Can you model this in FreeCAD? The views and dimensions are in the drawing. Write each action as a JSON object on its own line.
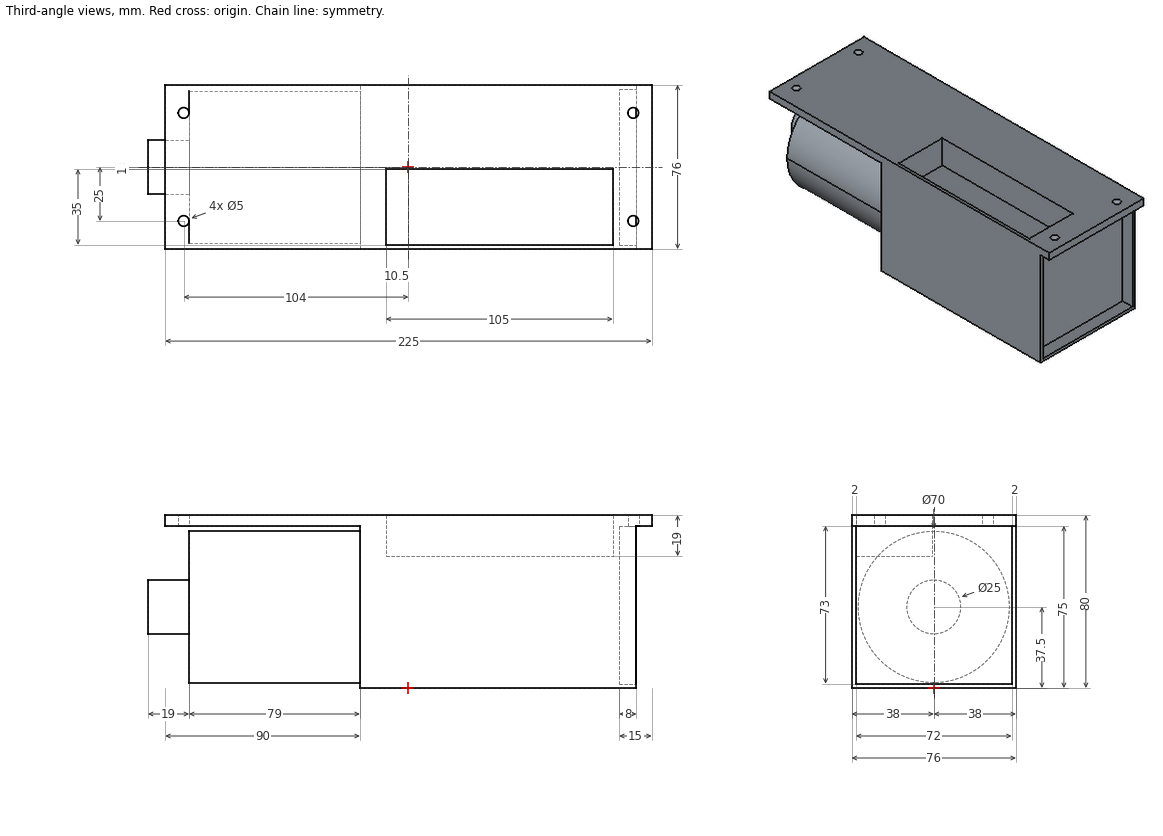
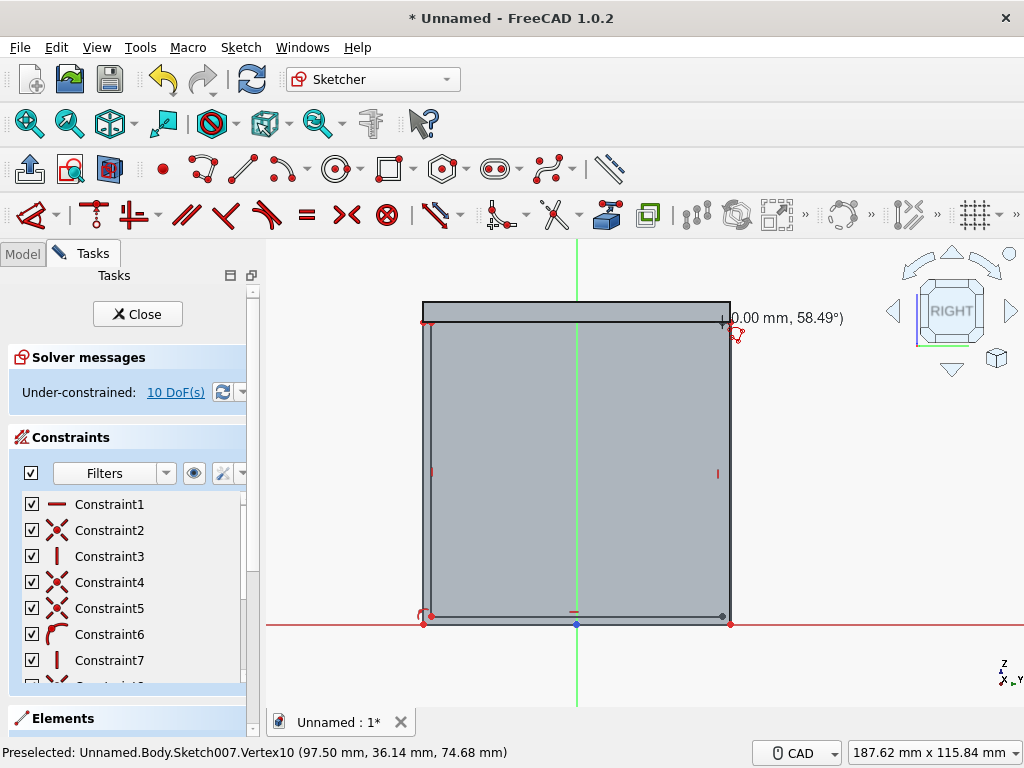
{"action": "scroll", "coordinate": [722, 617], "scroll_direction": "up", "scroll_amount": 4}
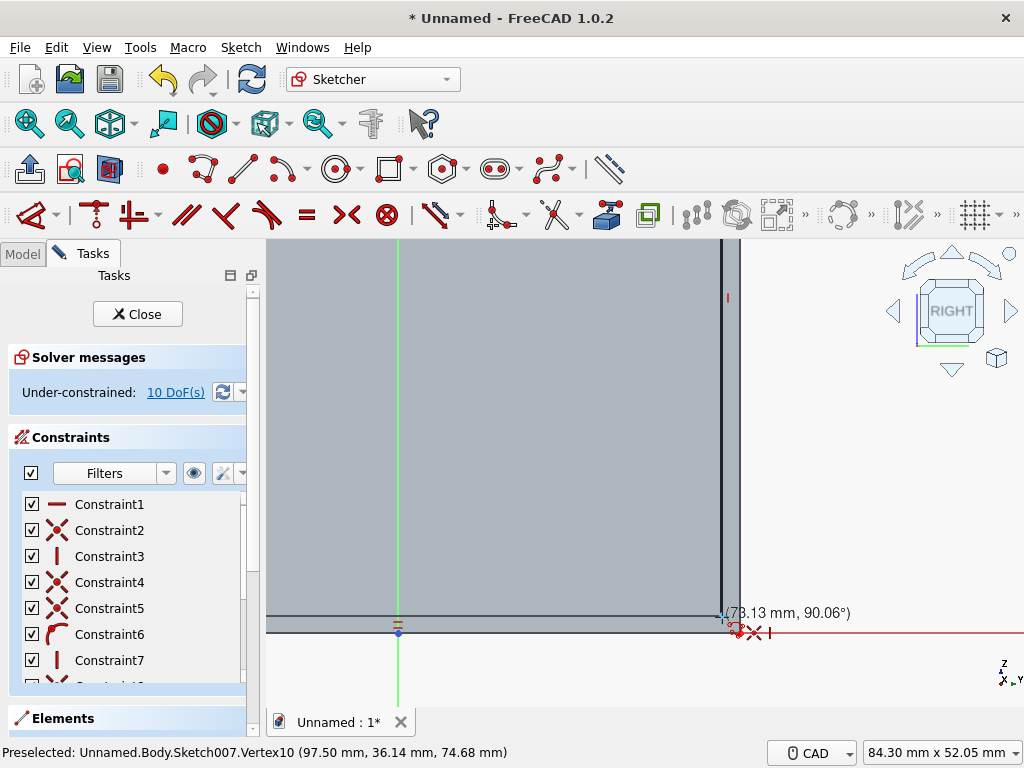
{"action": "left_click", "coordinate": [722, 616]}
{"action": "key", "text": "Escape"}
{"action": "key", "text": "Escape"}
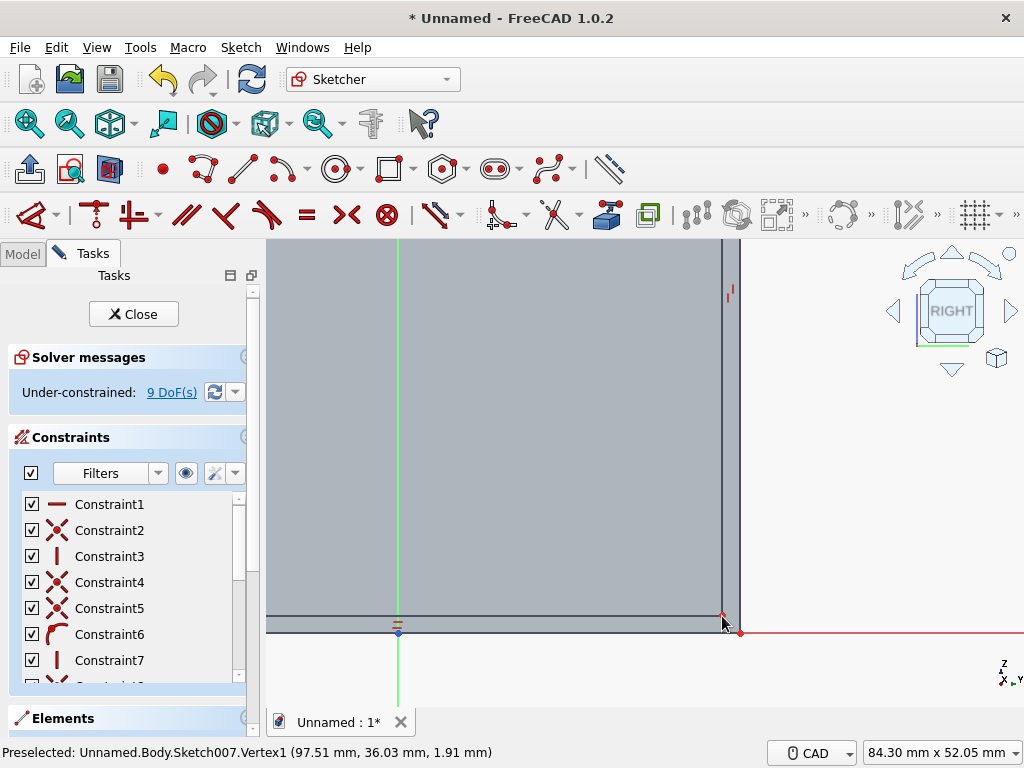
{"action": "scroll", "coordinate": [722, 617], "scroll_direction": "down", "scroll_amount": 4}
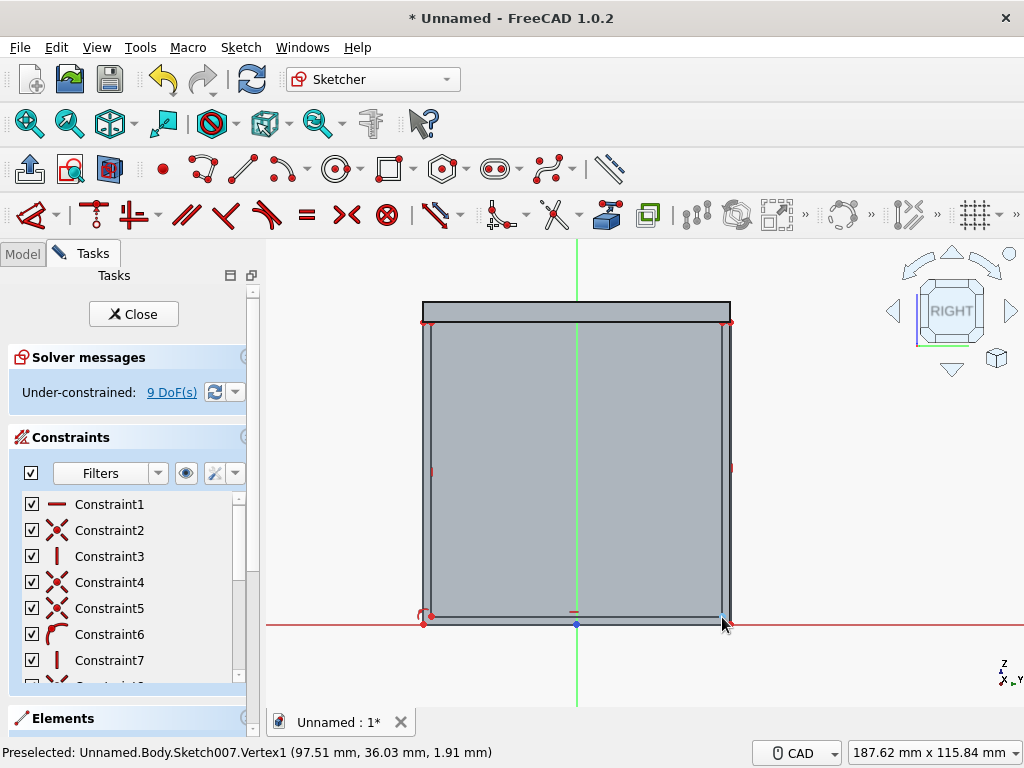
{"action": "scroll", "coordinate": [427, 323], "scroll_direction": "up", "scroll_amount": 7}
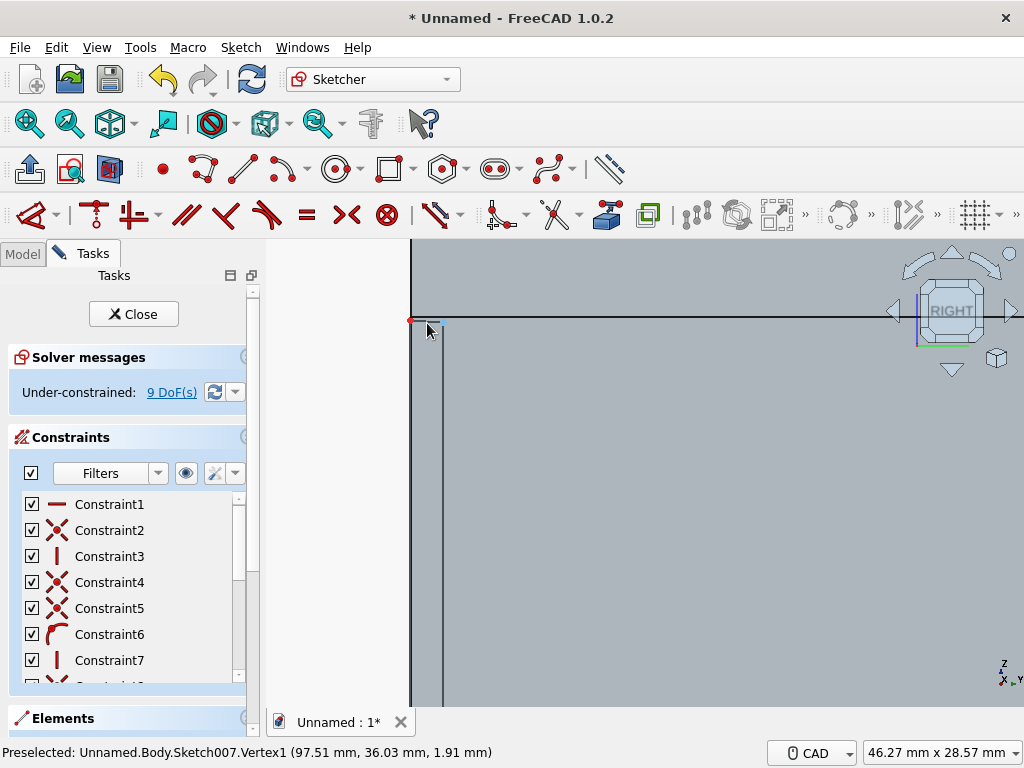
{"action": "left_click", "coordinate": [427, 322]}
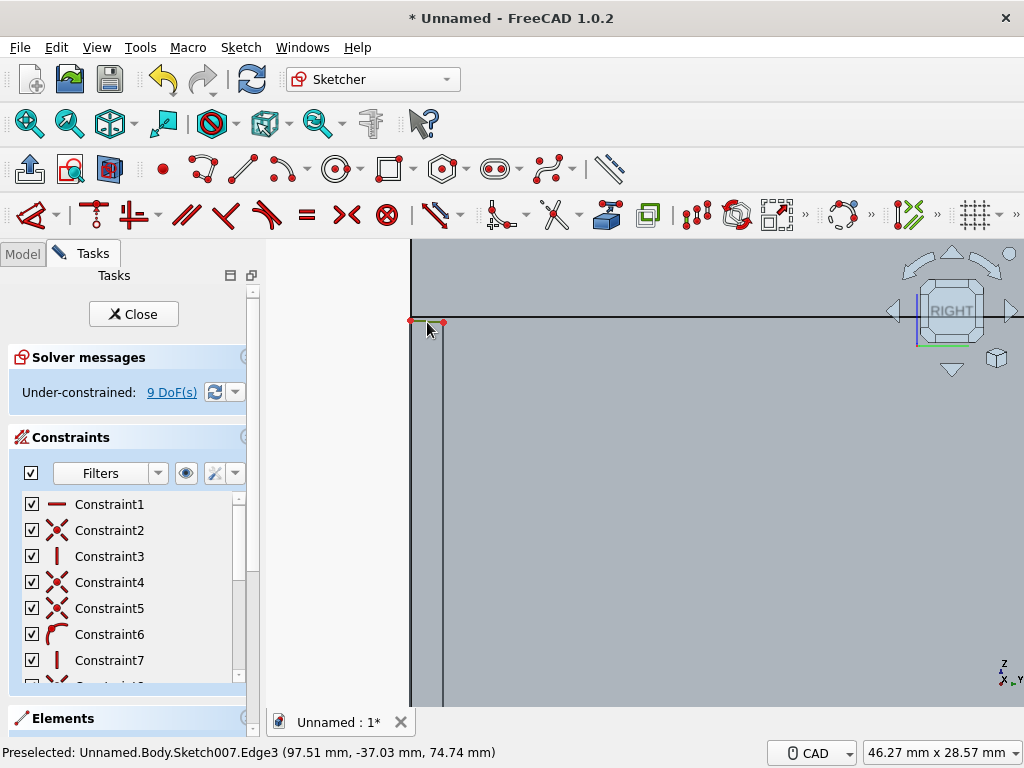
{"action": "key", "text": "h"}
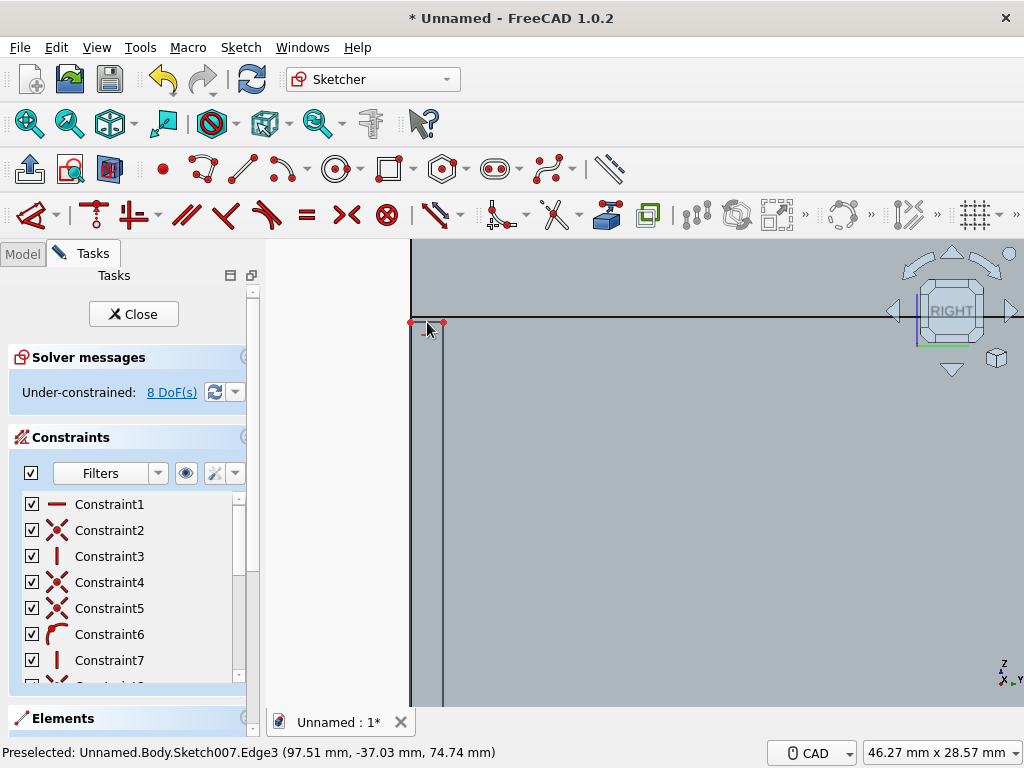
{"action": "scroll", "coordinate": [427, 323], "scroll_direction": "down", "scroll_amount": 7}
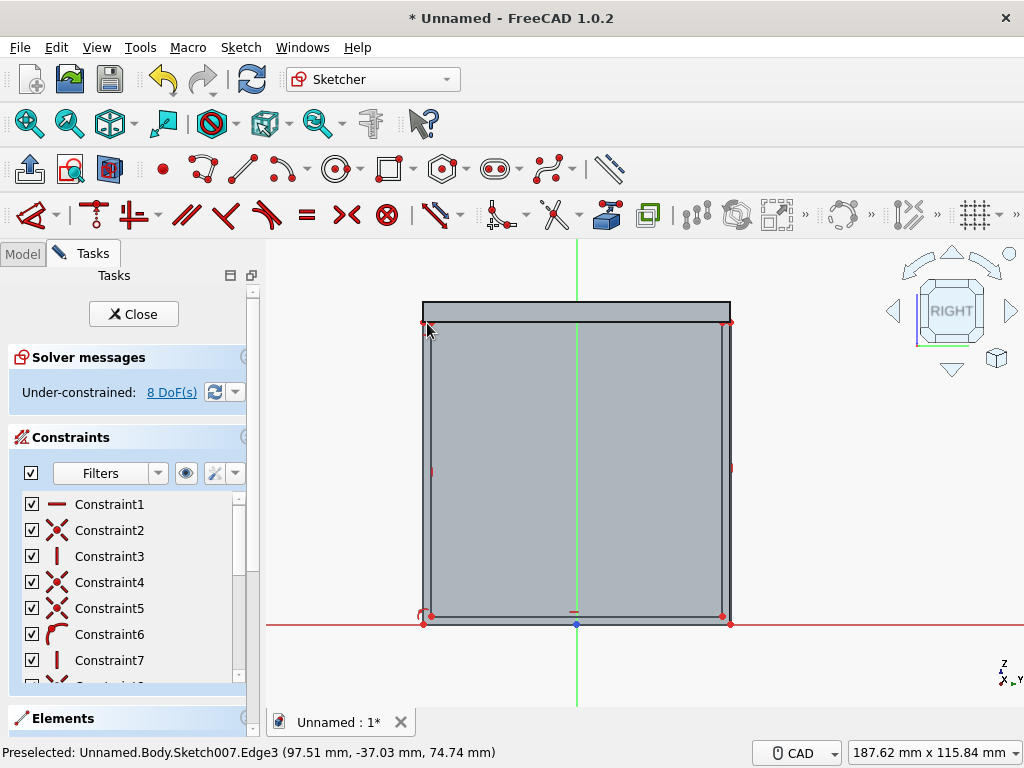
{"action": "scroll", "coordinate": [728, 323], "scroll_direction": "up", "scroll_amount": 9}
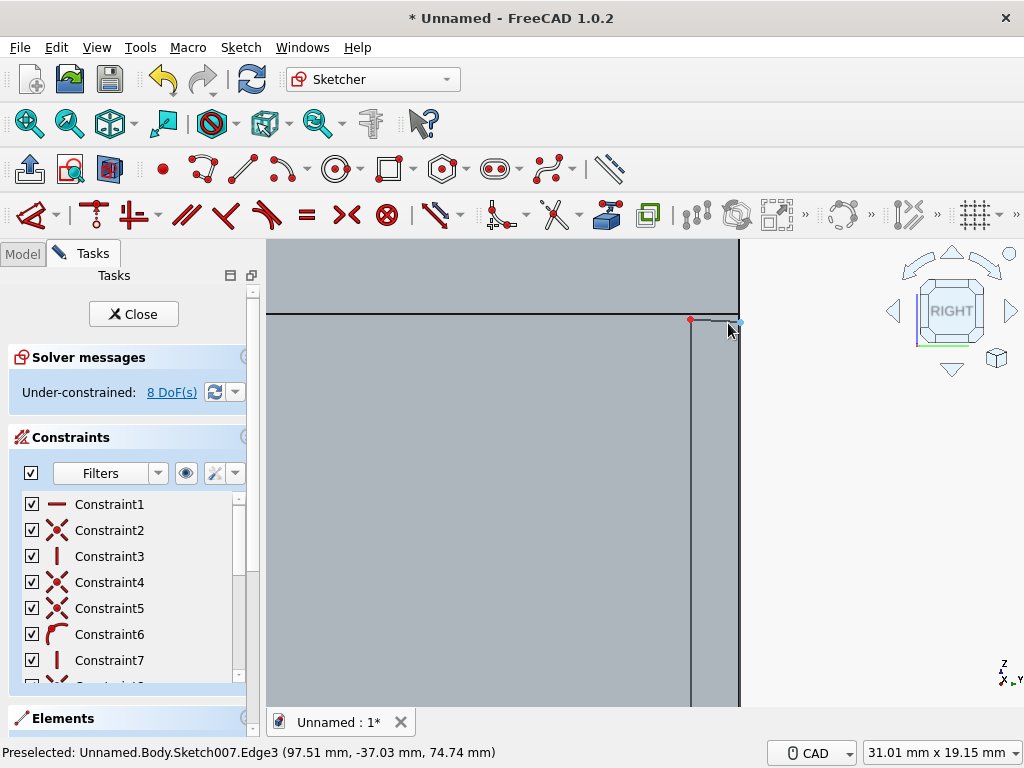
{"action": "left_click", "coordinate": [725, 321]}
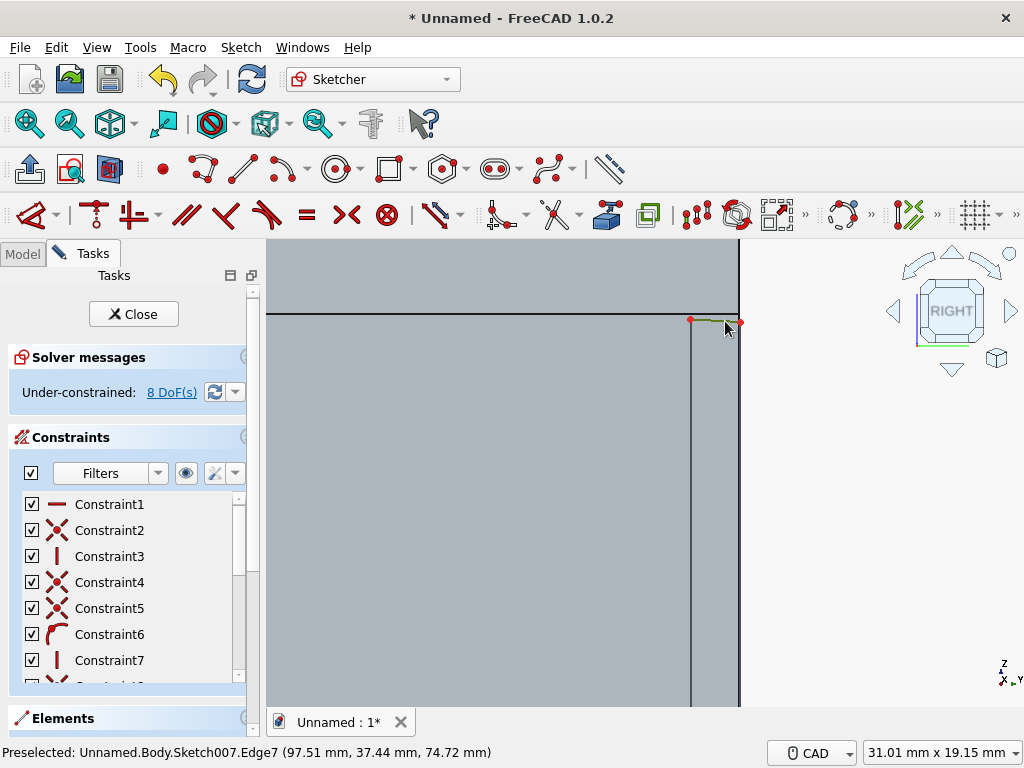
{"action": "key", "text": "h"}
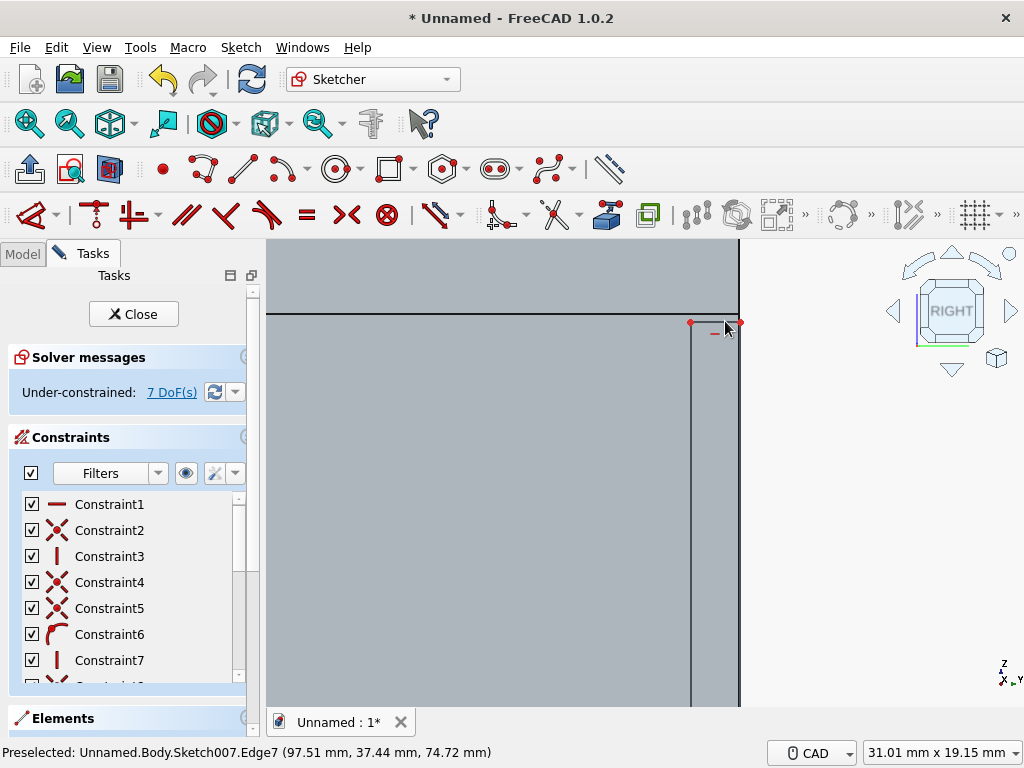
{"action": "scroll", "coordinate": [728, 323], "scroll_direction": "down", "scroll_amount": 9}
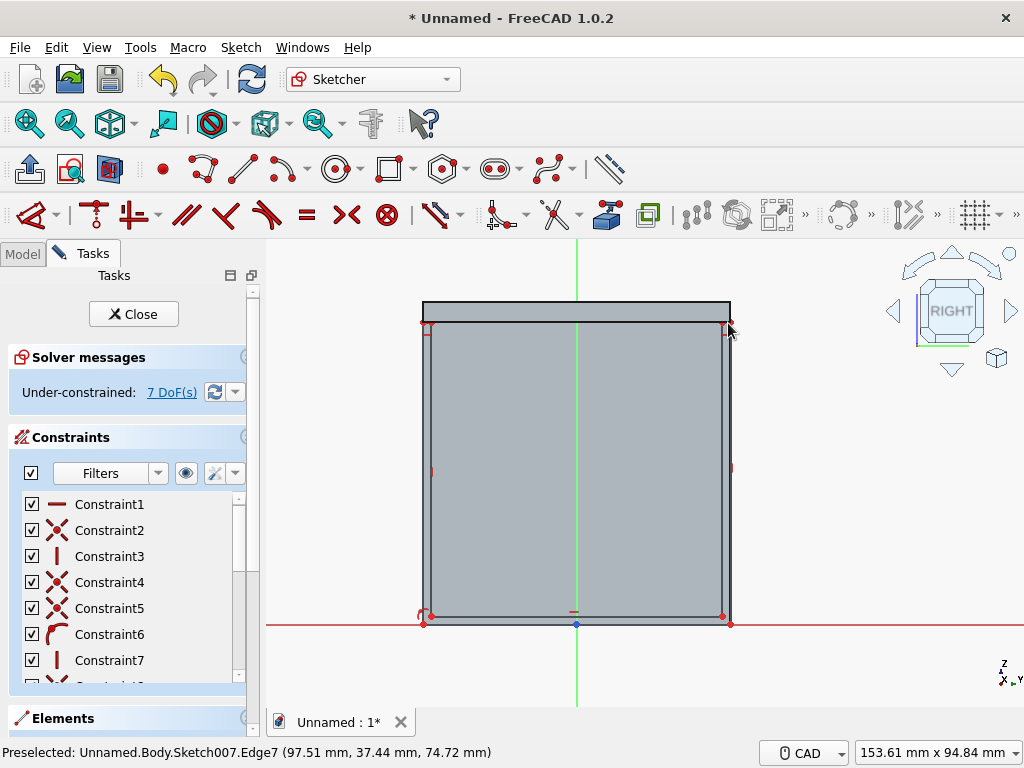
{"action": "scroll", "coordinate": [423, 323], "scroll_direction": "up", "scroll_amount": 3}